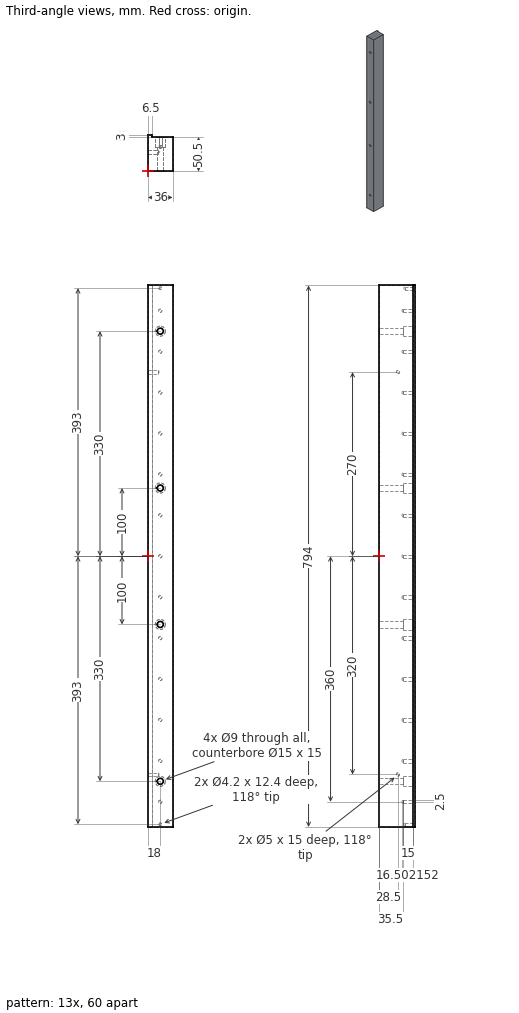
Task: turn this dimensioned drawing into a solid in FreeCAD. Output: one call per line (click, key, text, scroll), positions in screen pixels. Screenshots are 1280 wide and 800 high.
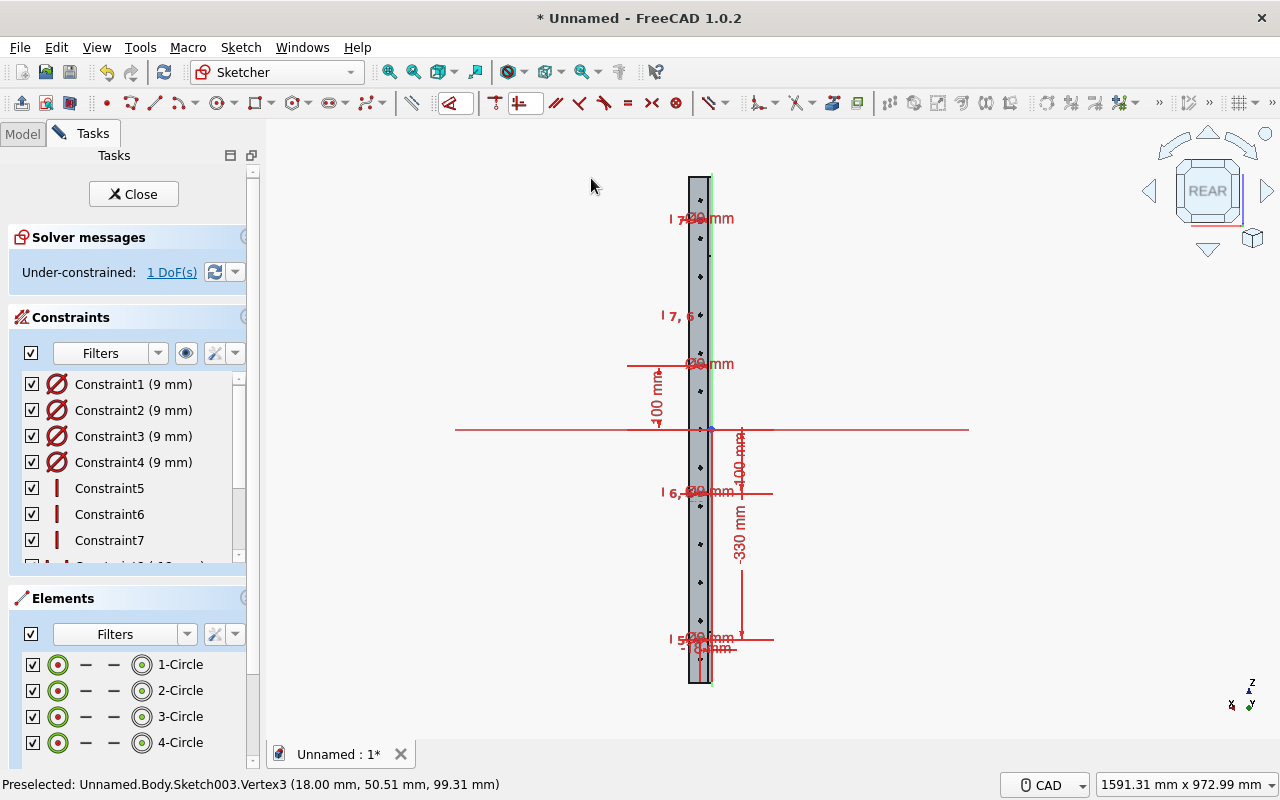
click(700, 220)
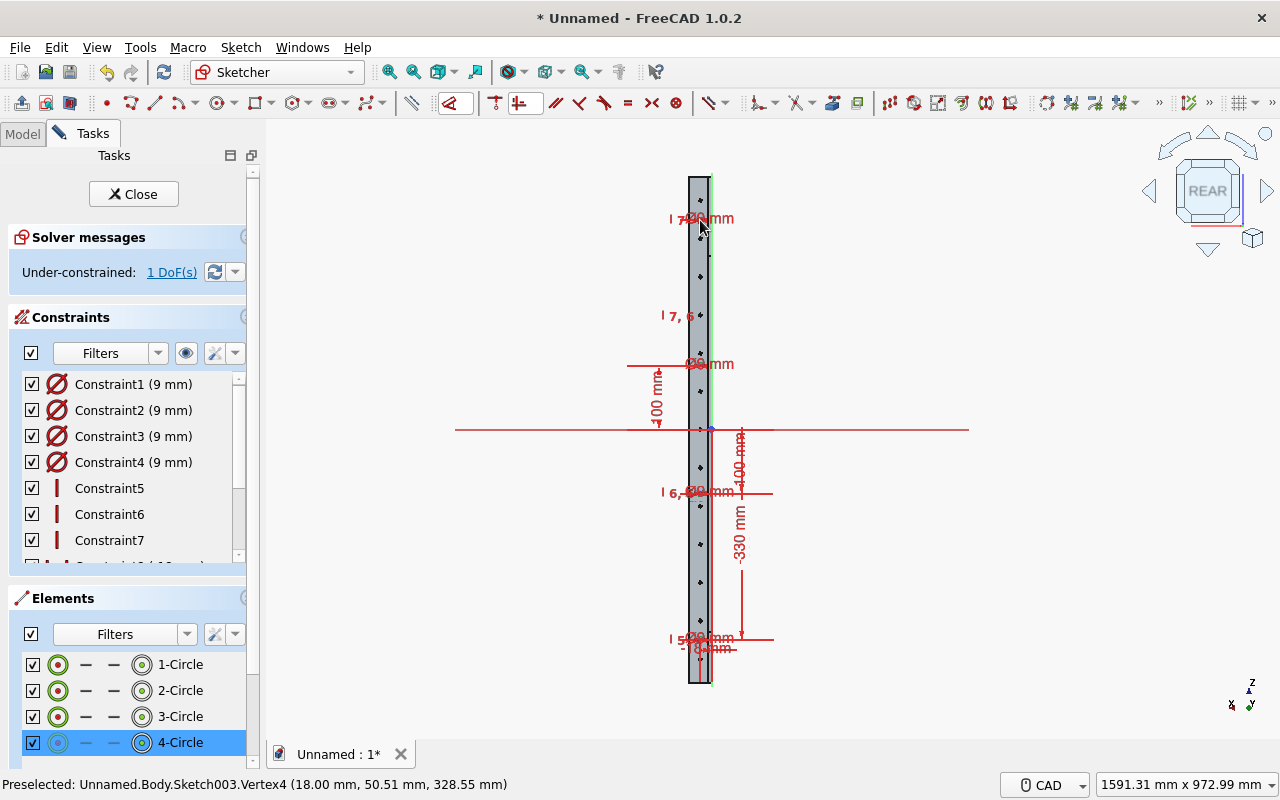
click(468, 104)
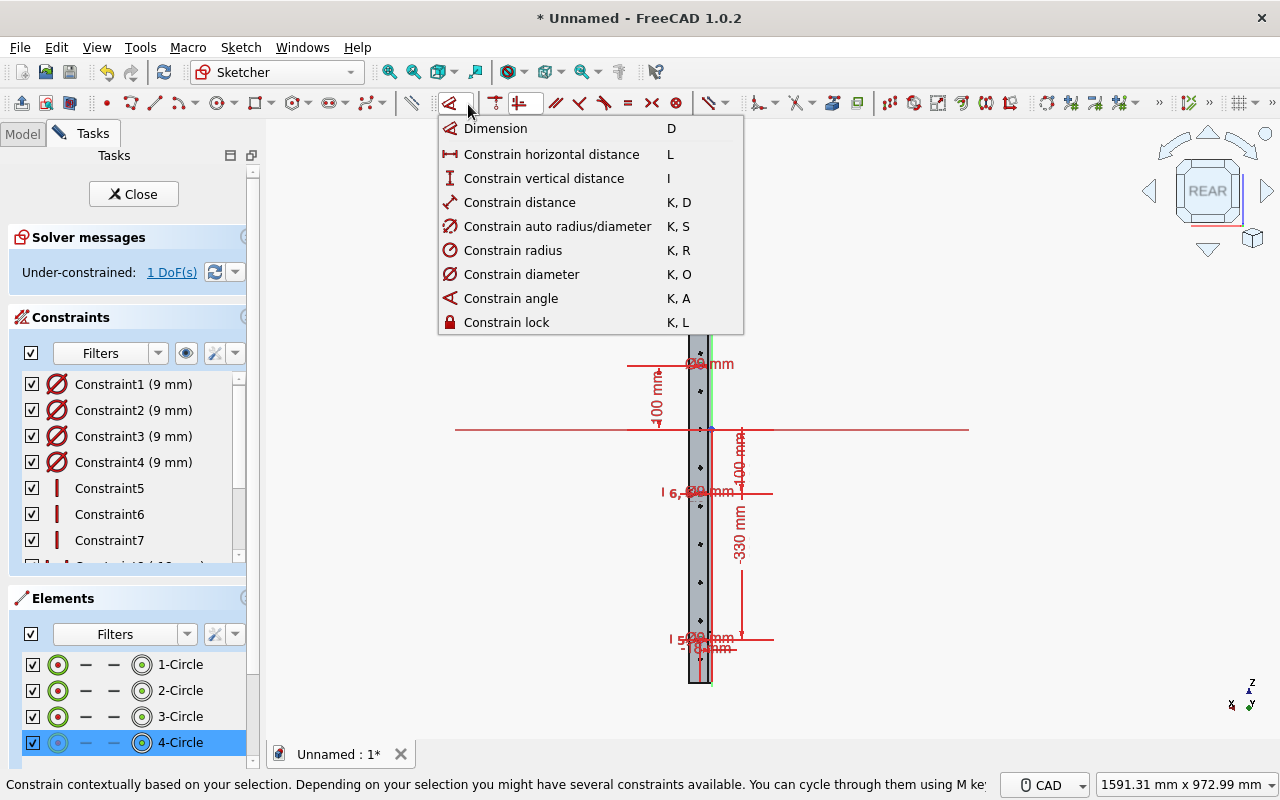
click(591, 178)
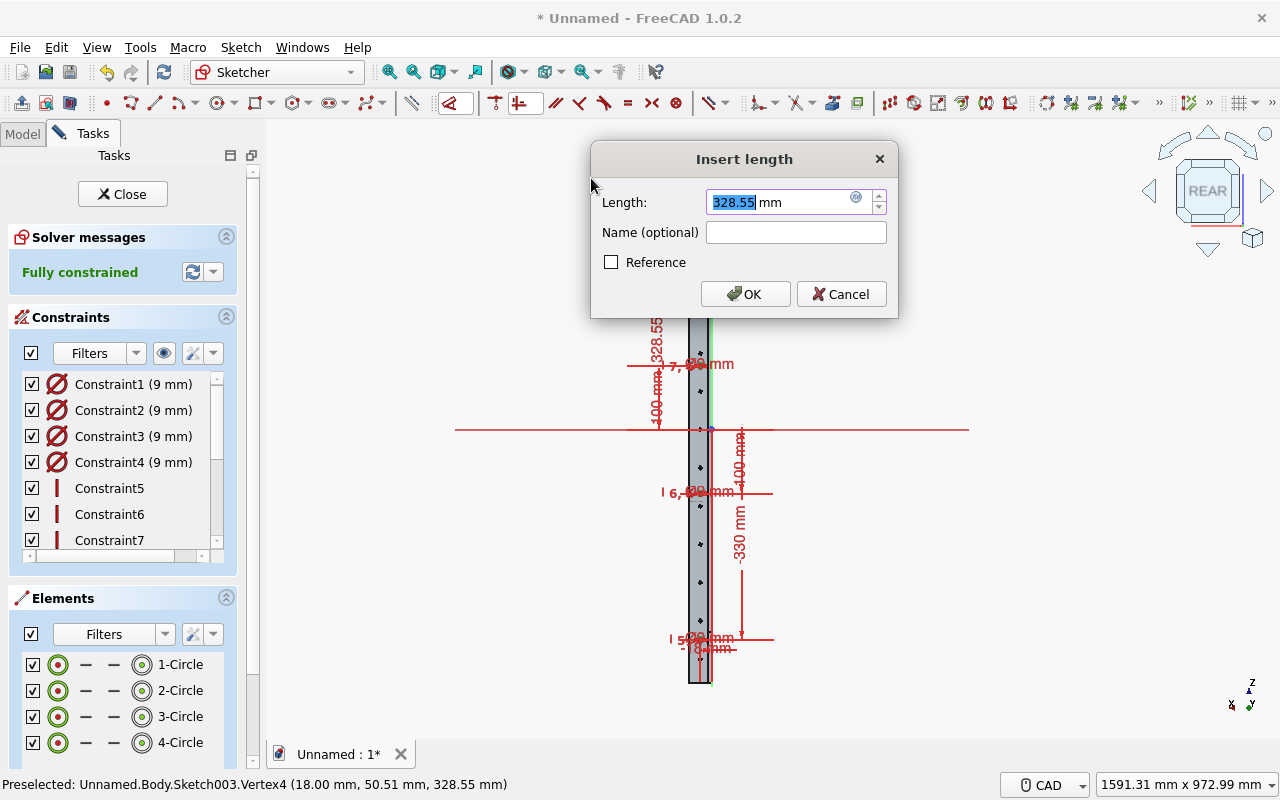
text(330)
key(Return)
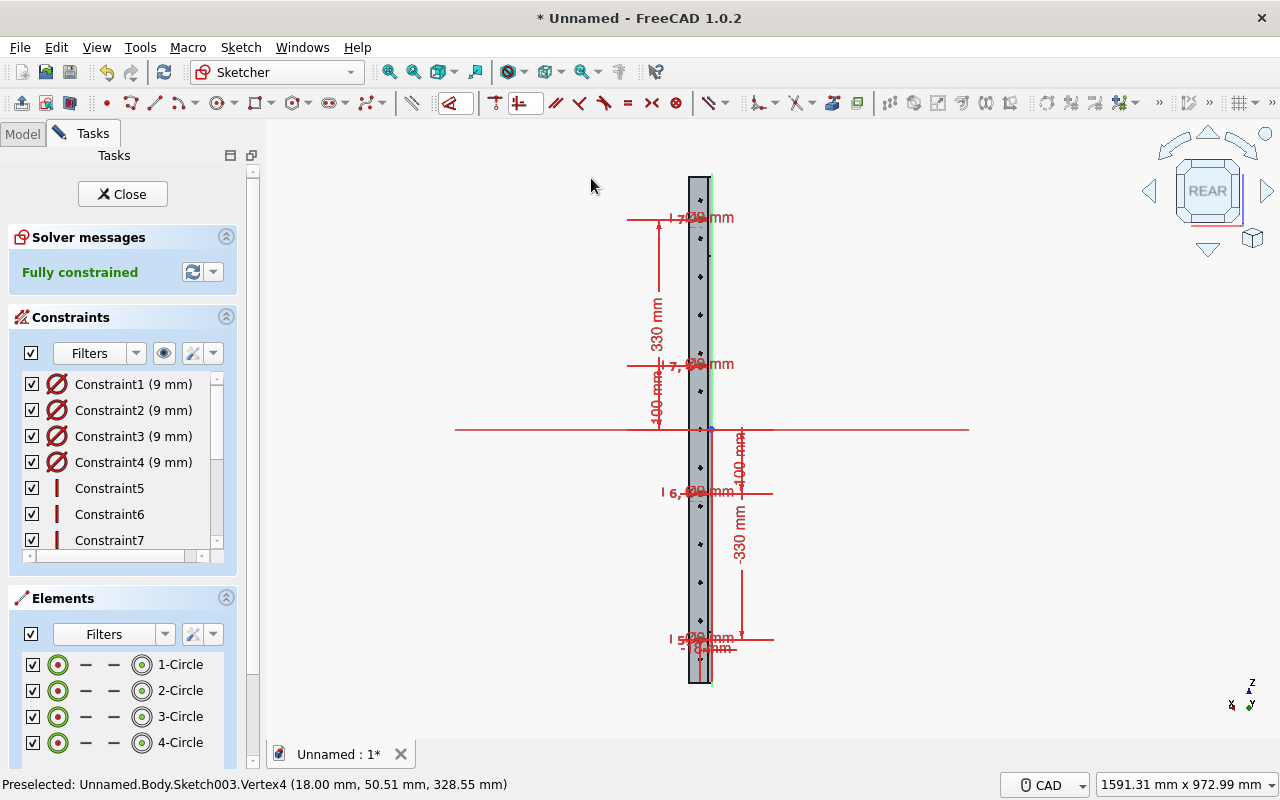
click(123, 194)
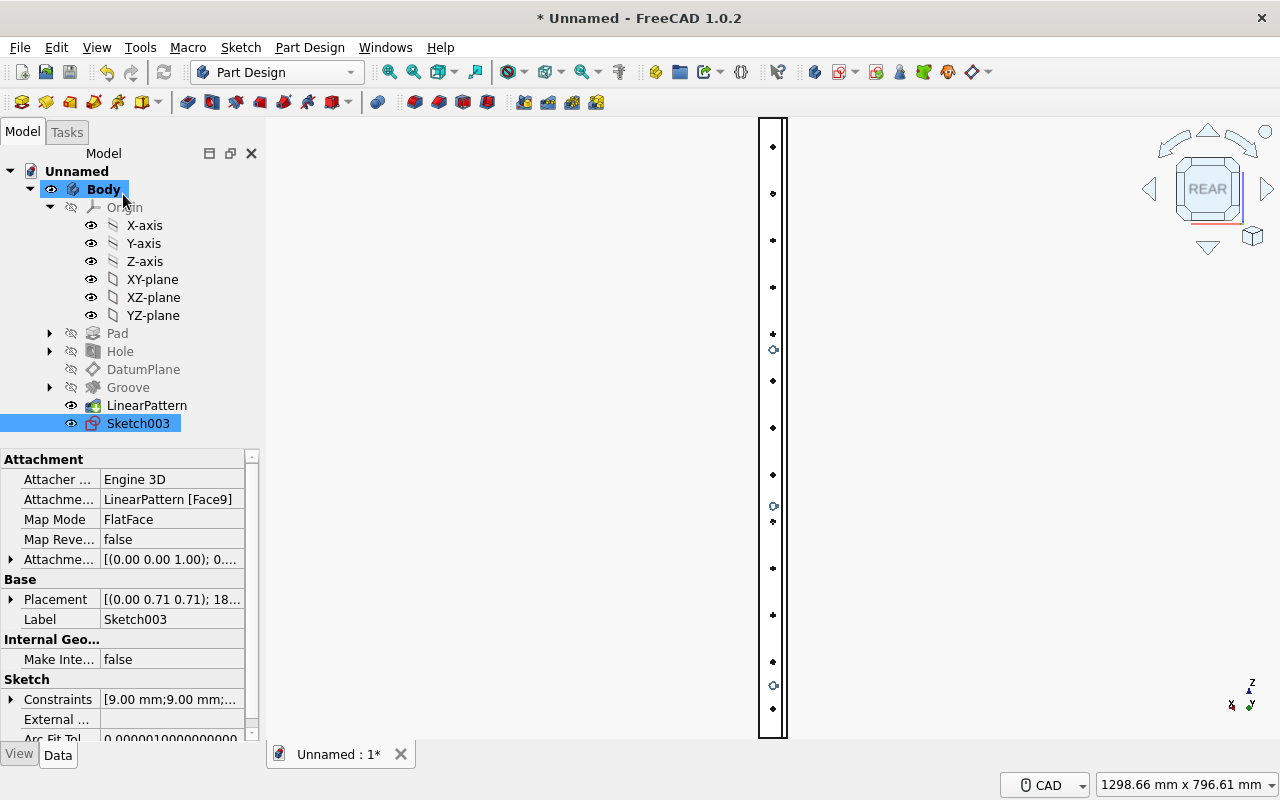
click(212, 102)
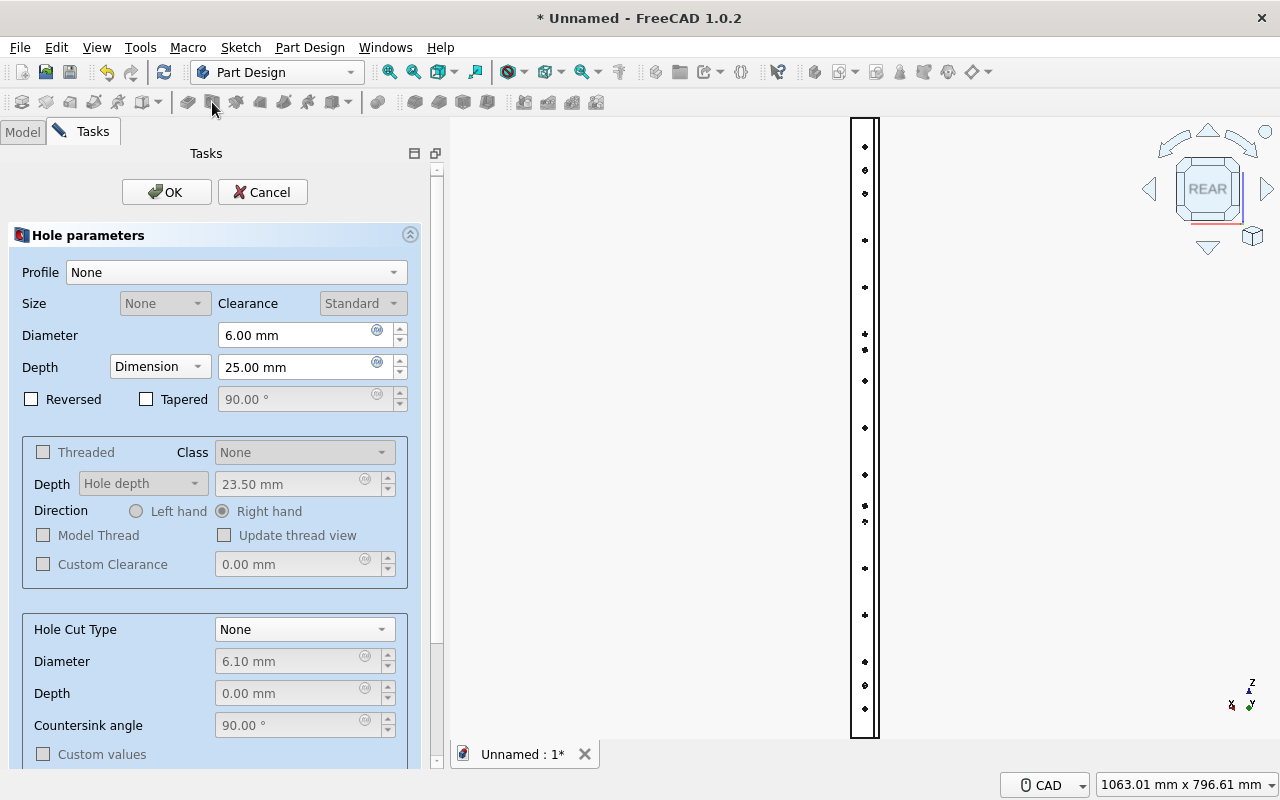
triple_click(305, 335)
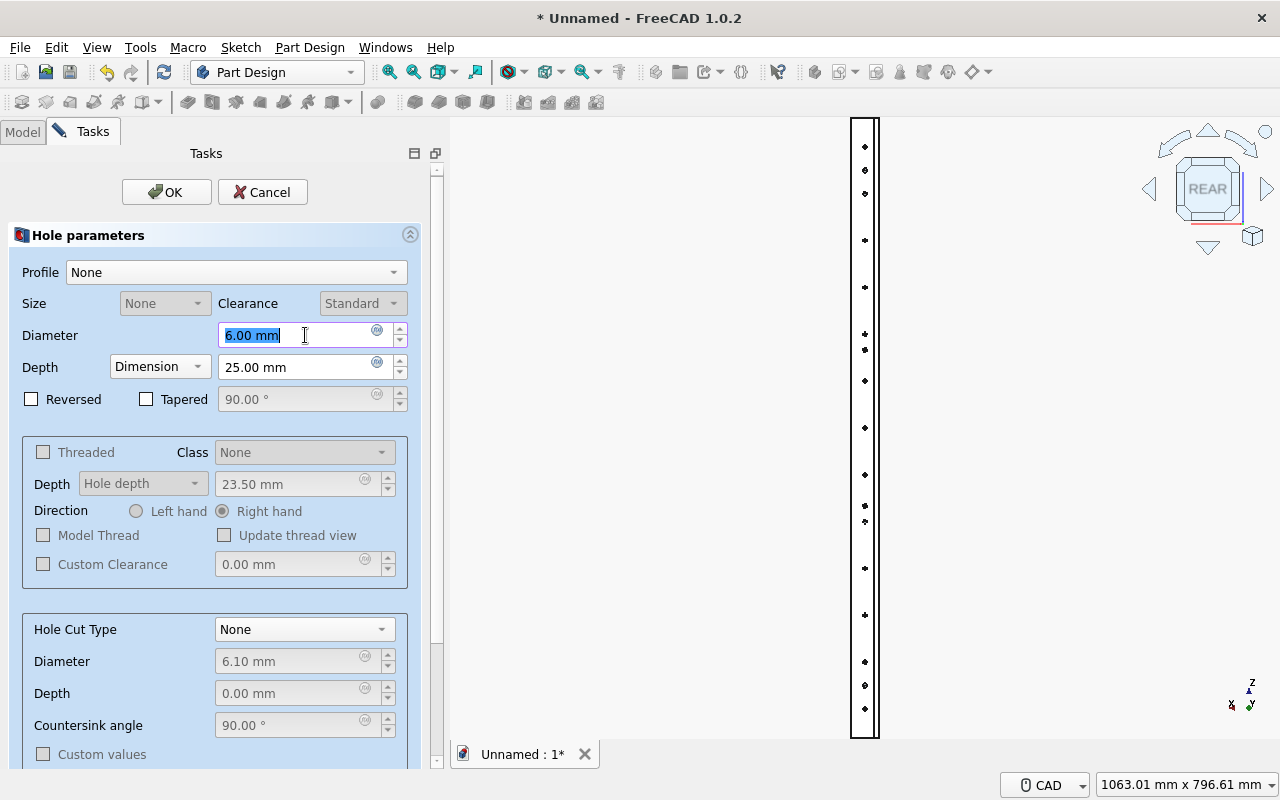
text(9)
key(Tab)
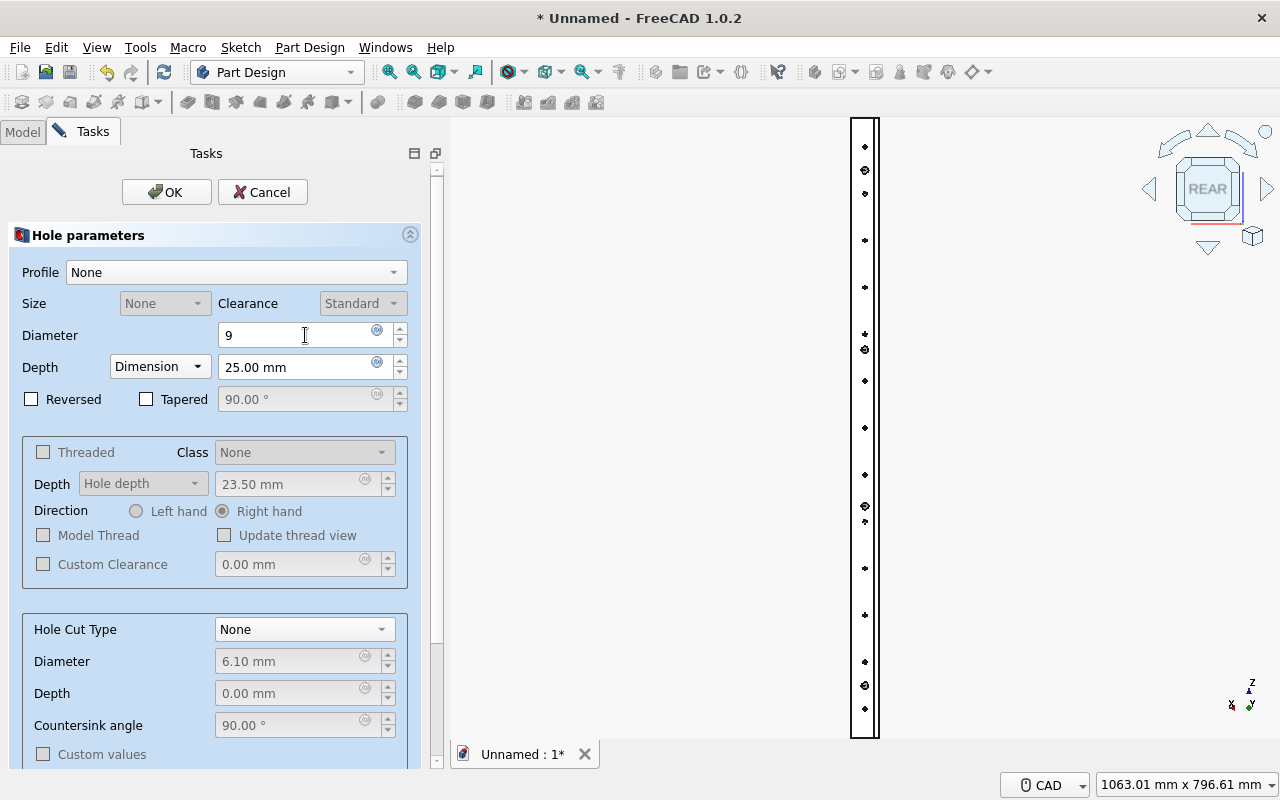
click(161, 366)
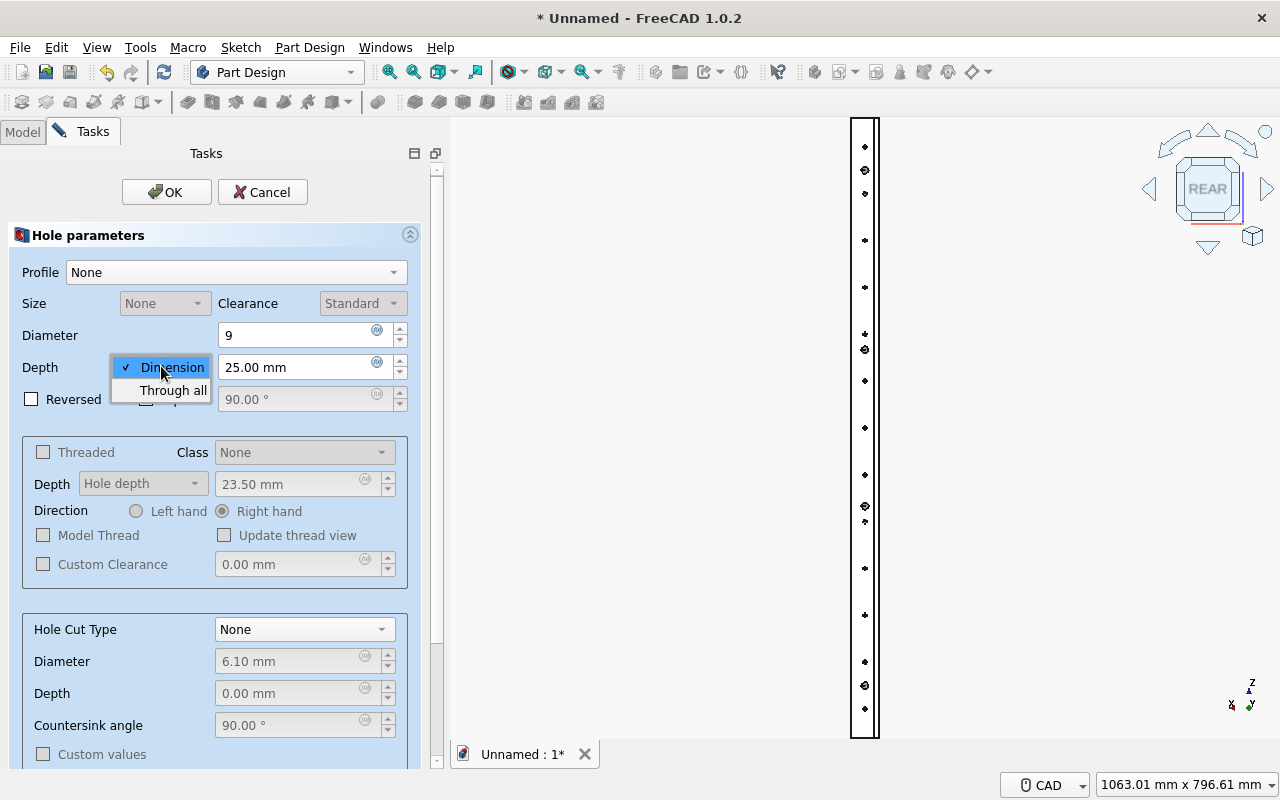
click(160, 390)